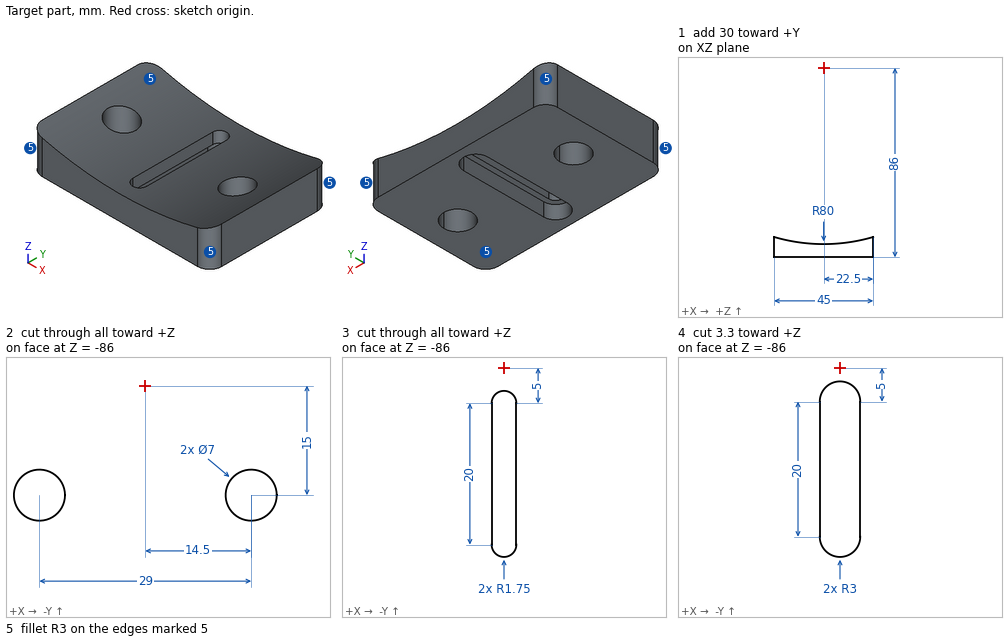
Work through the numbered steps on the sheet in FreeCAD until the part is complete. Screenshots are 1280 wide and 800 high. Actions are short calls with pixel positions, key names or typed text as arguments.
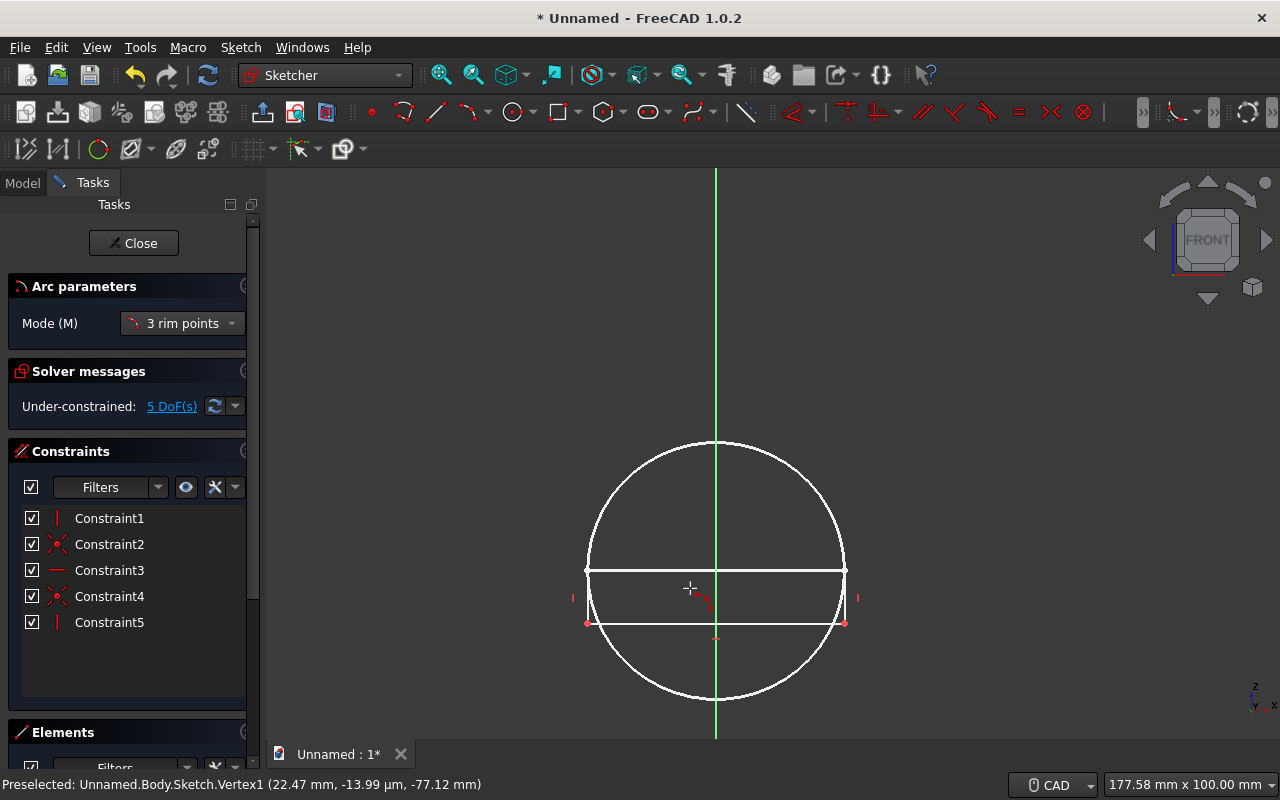
click(690, 587)
key(Escape)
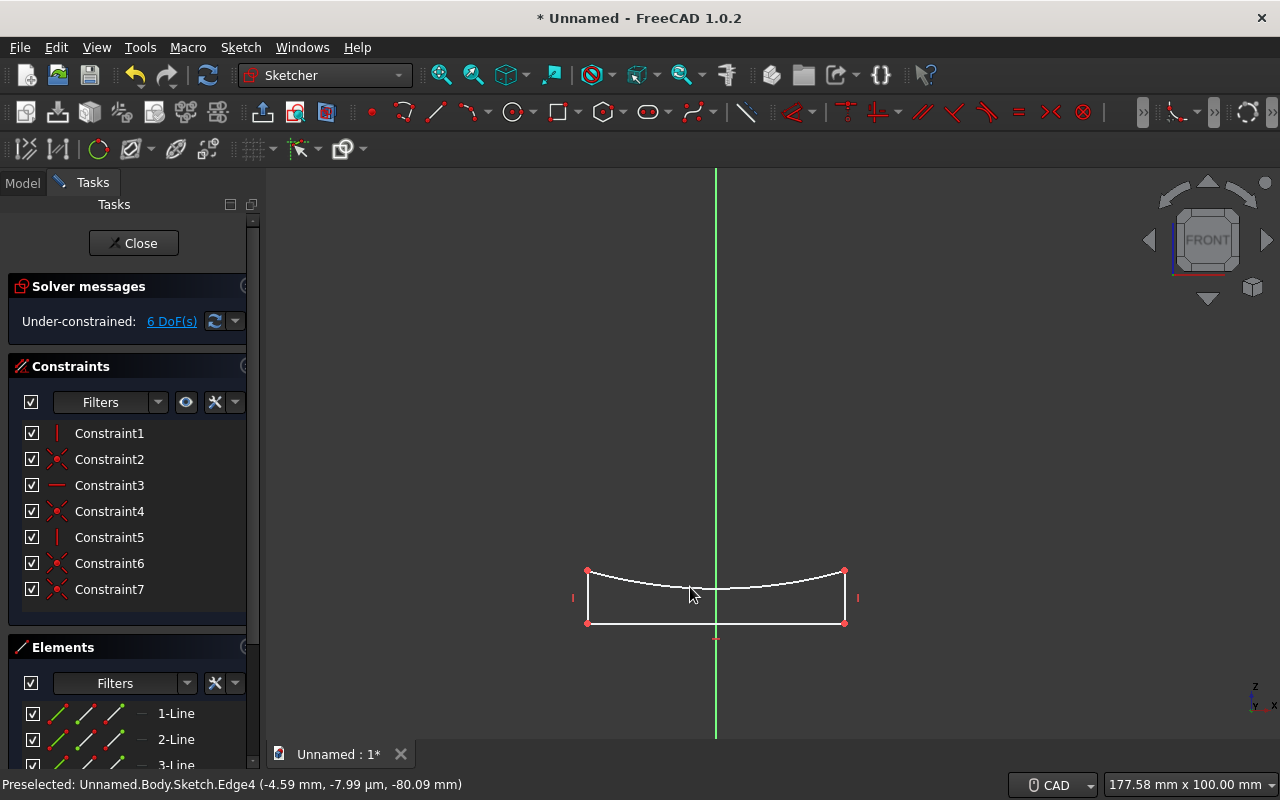
scroll(681, 611, down, 2)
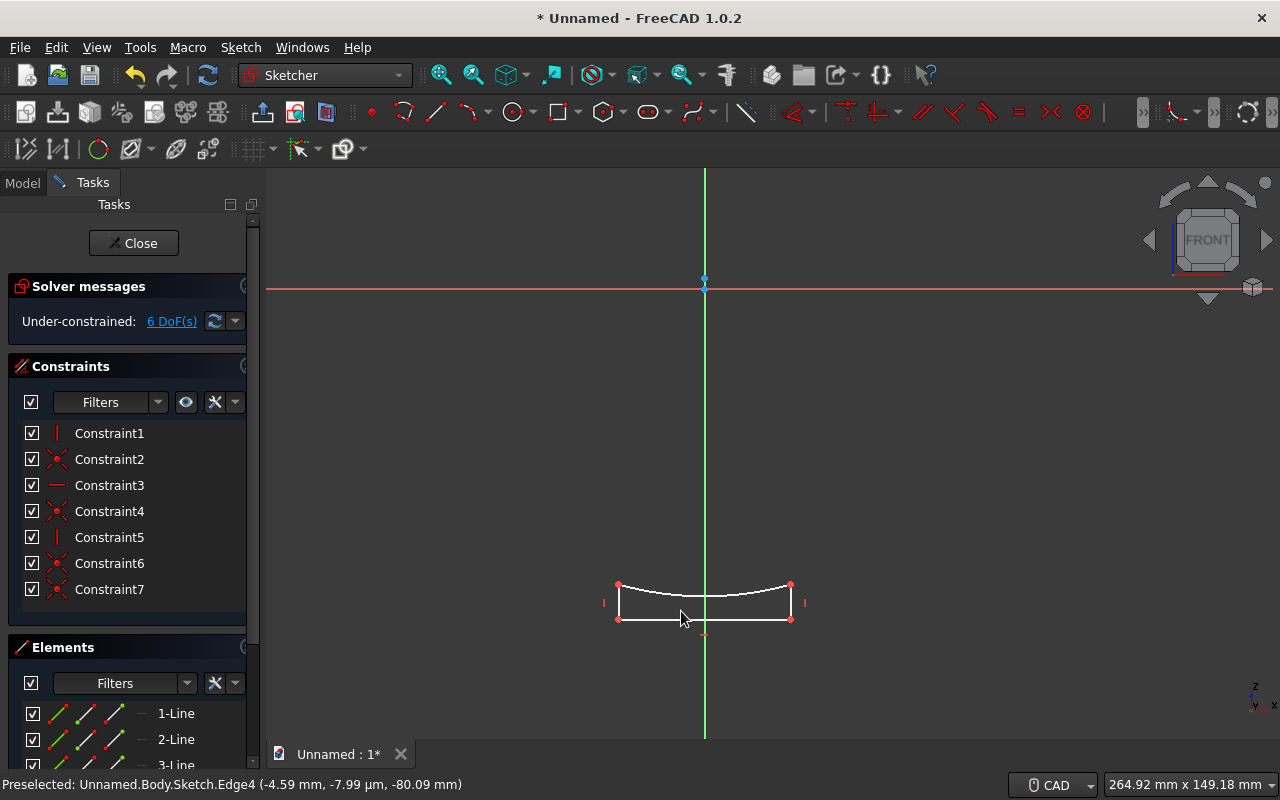
drag(695, 268, 715, 299)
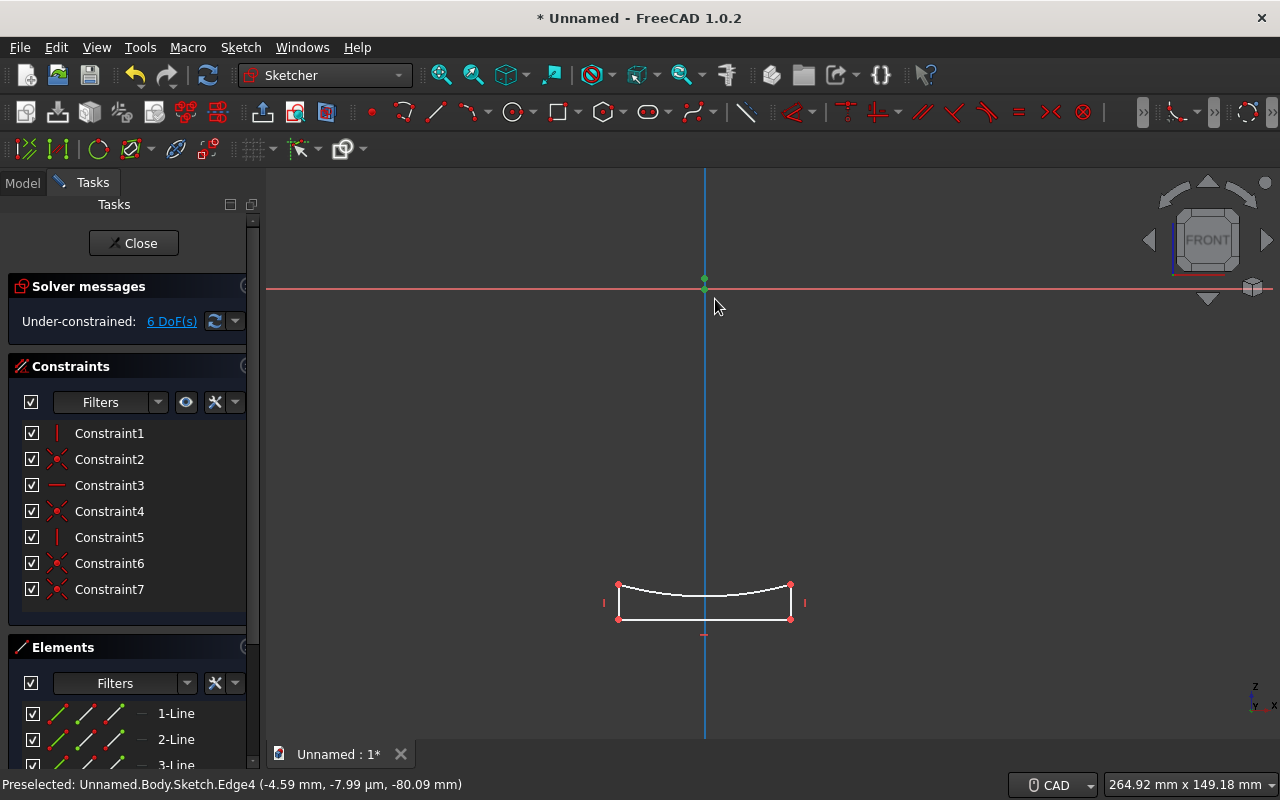
click(846, 112)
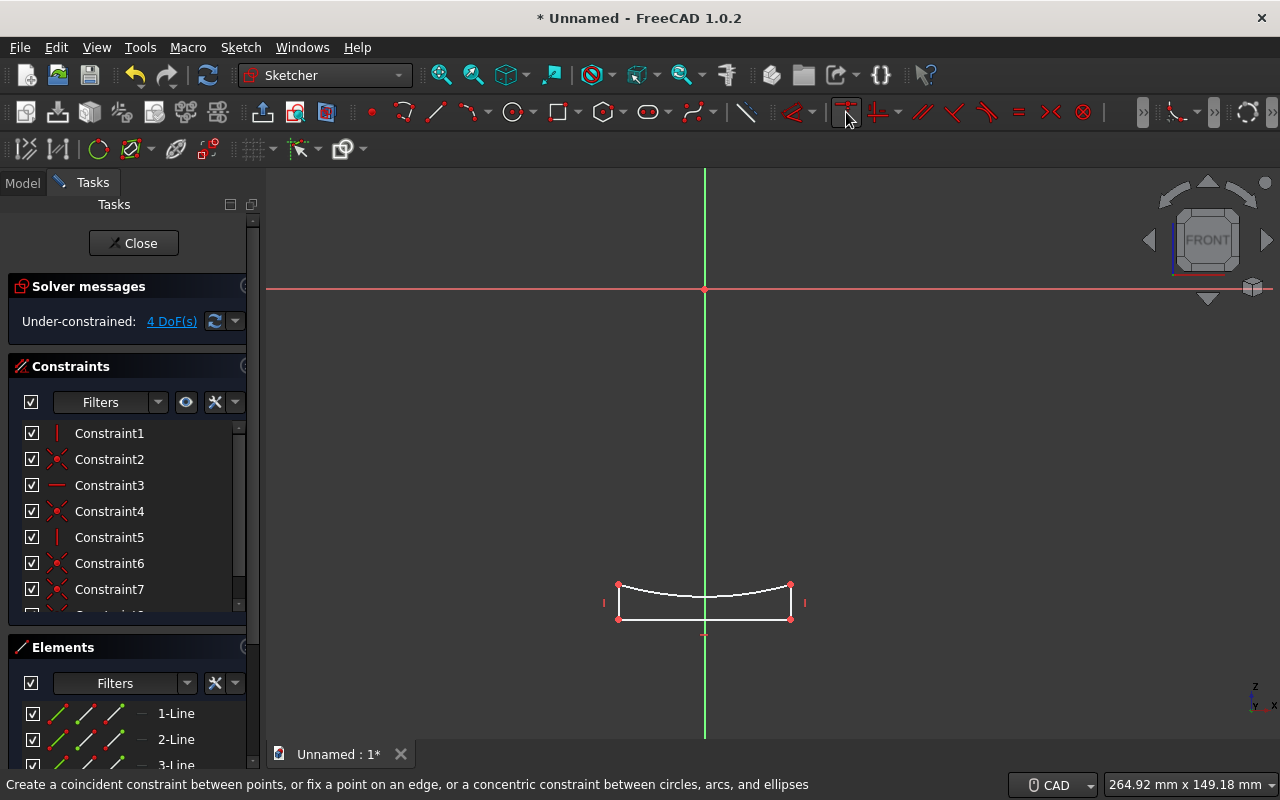
click(792, 112)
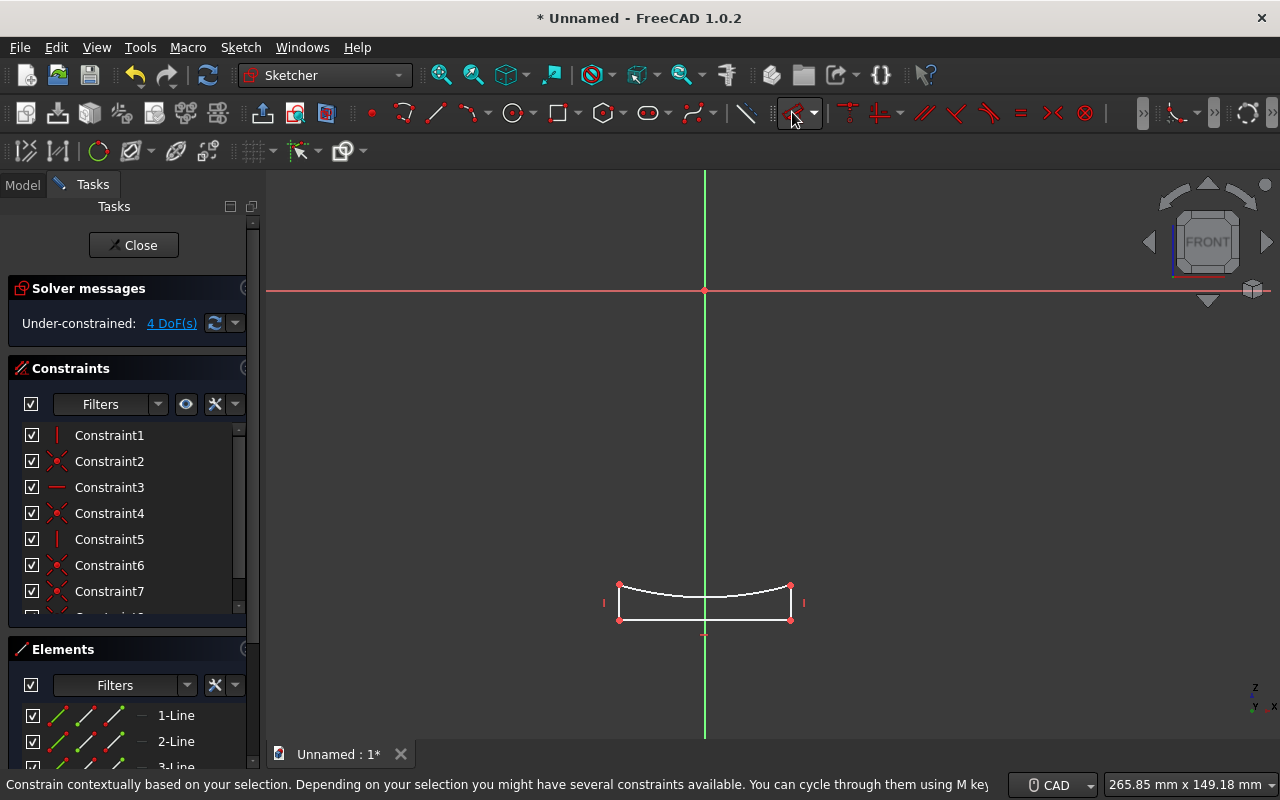
click(670, 595)
click(510, 567)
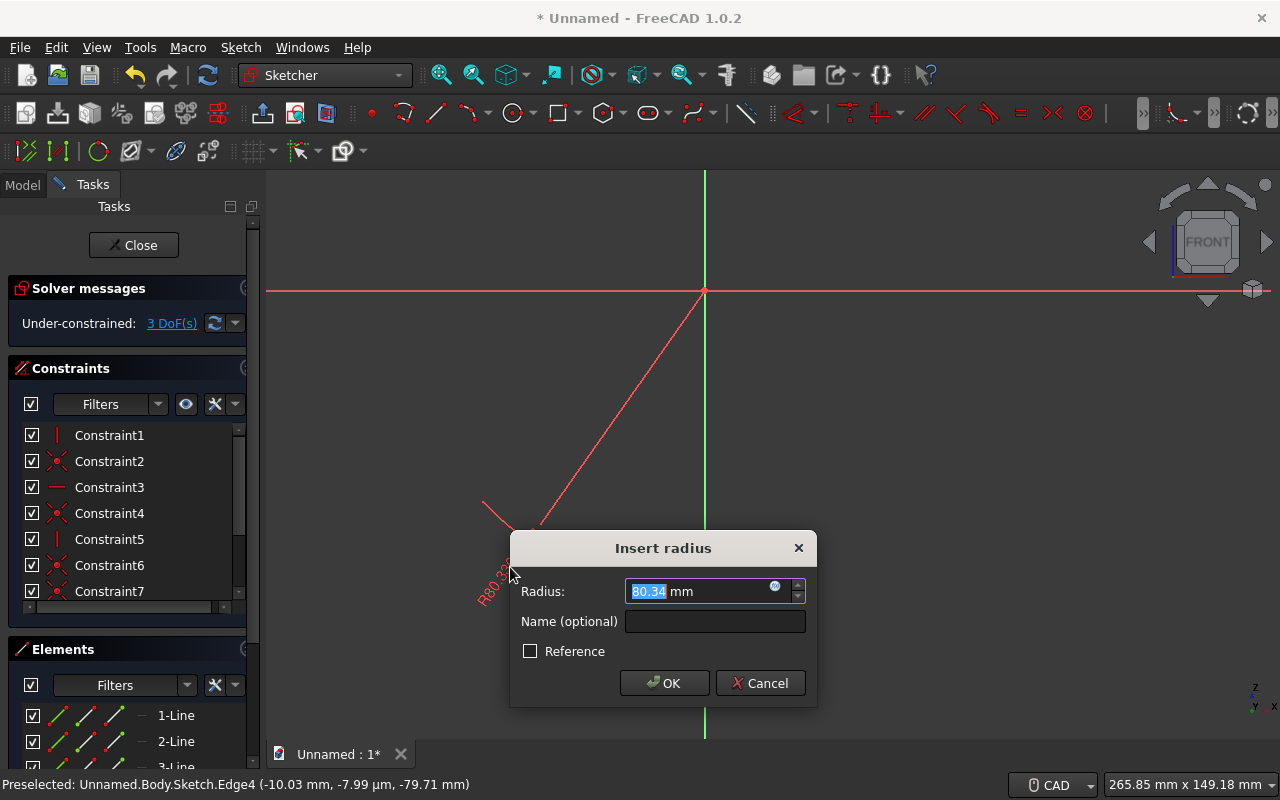
text(80)
key(Return)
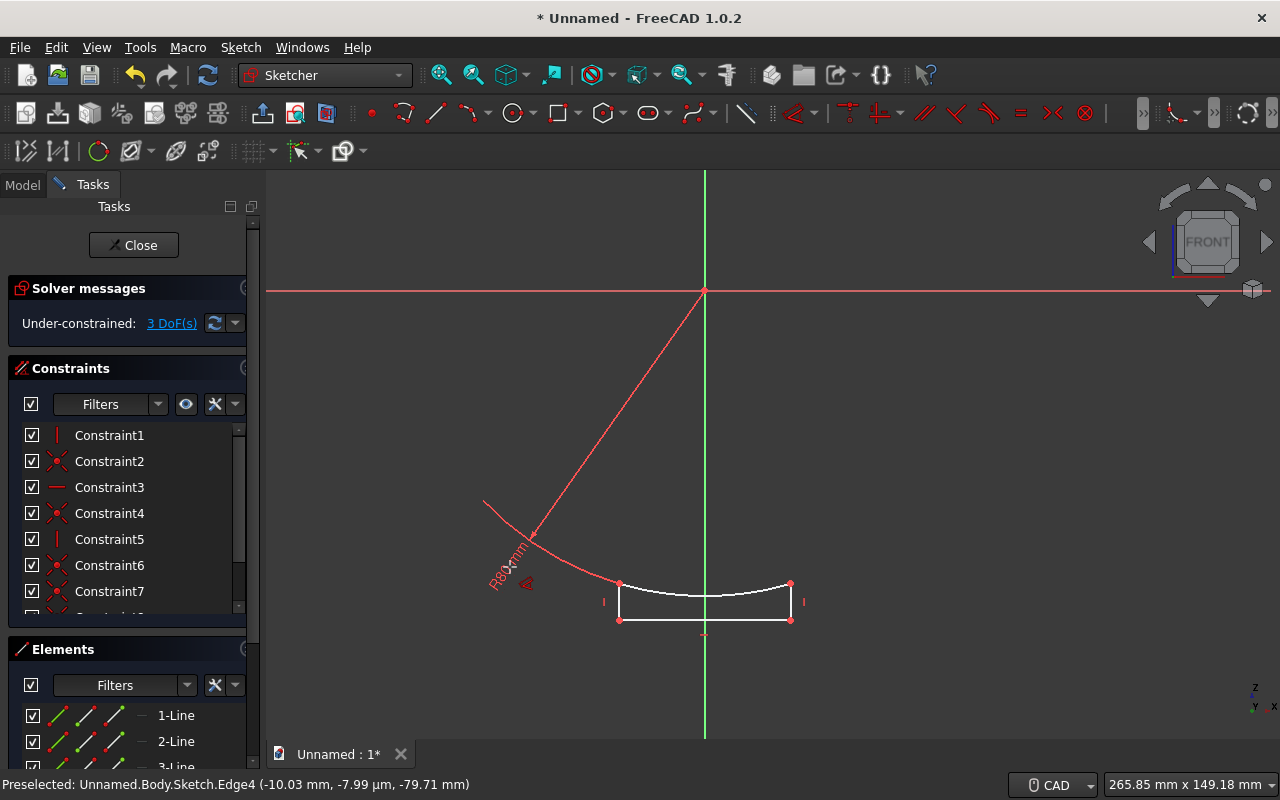
click(739, 620)
click(665, 654)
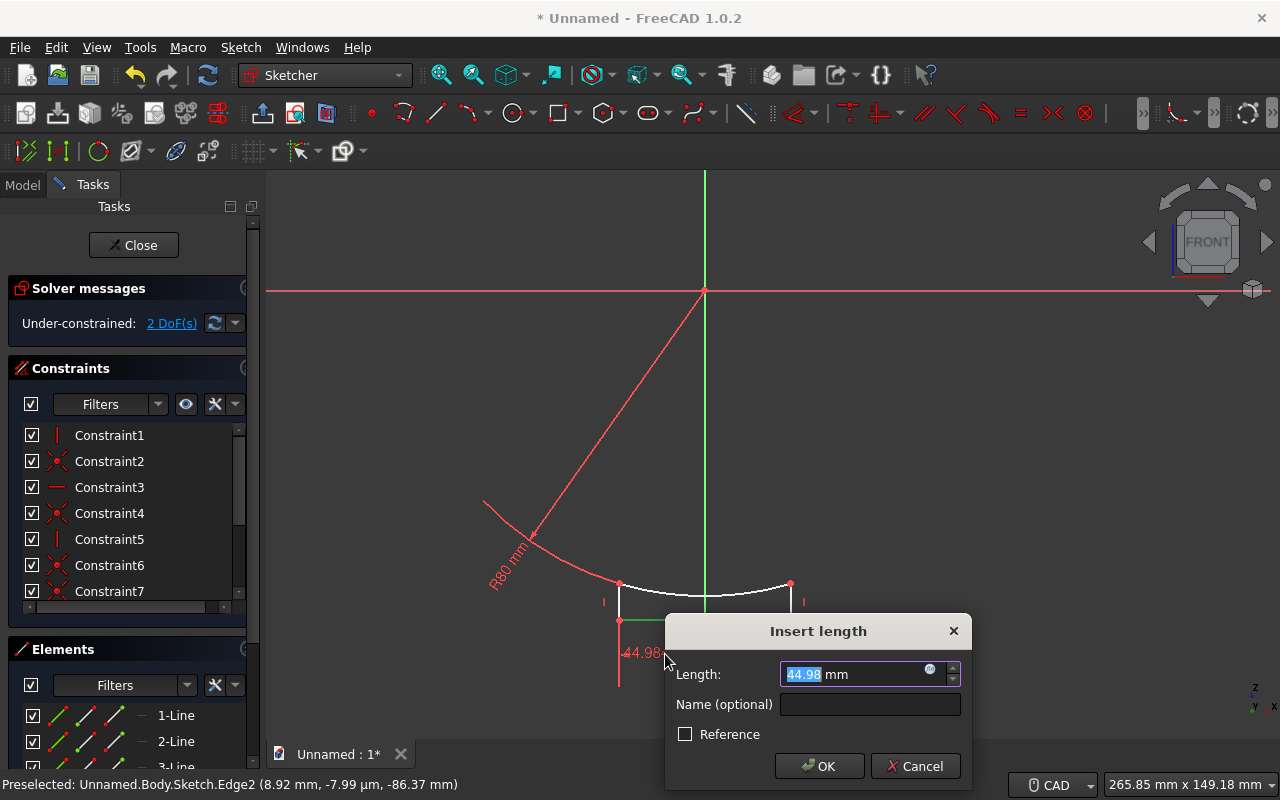
text(45)
key(Return)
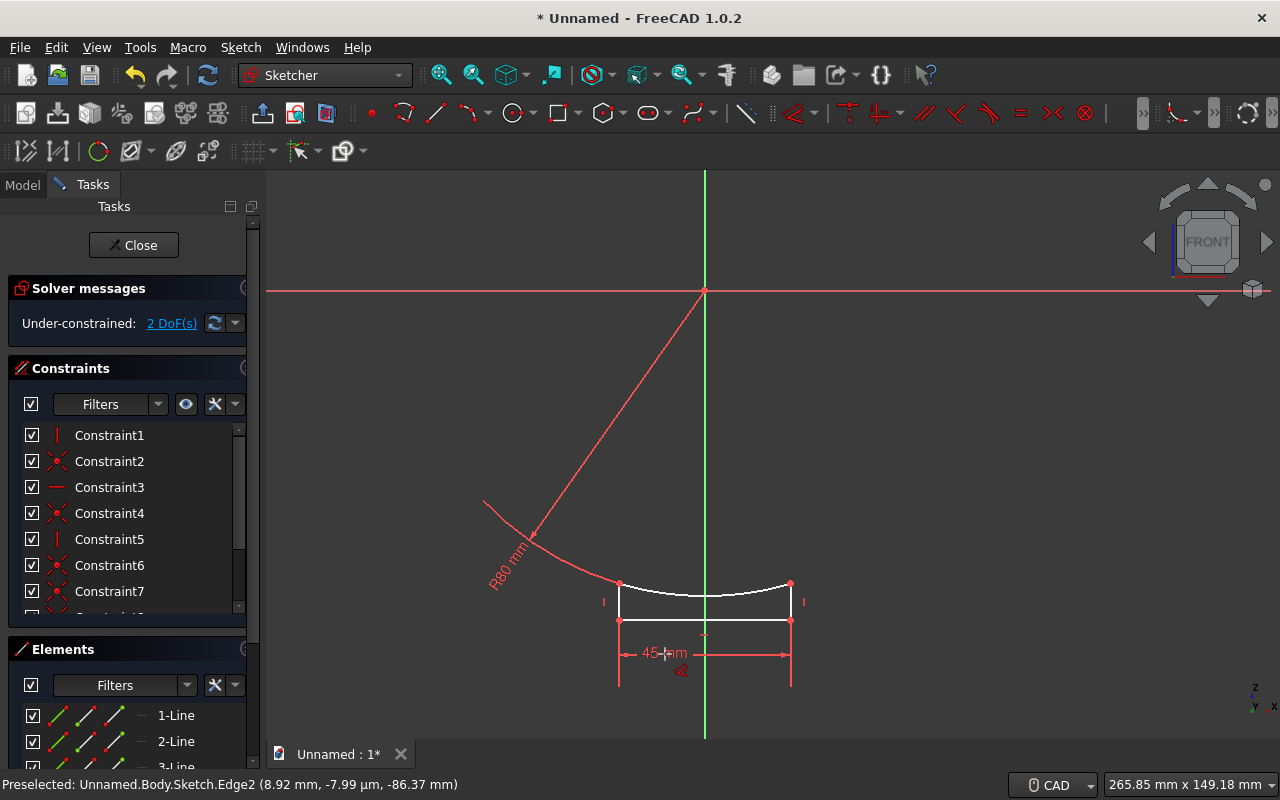
click(791, 620)
click(825, 456)